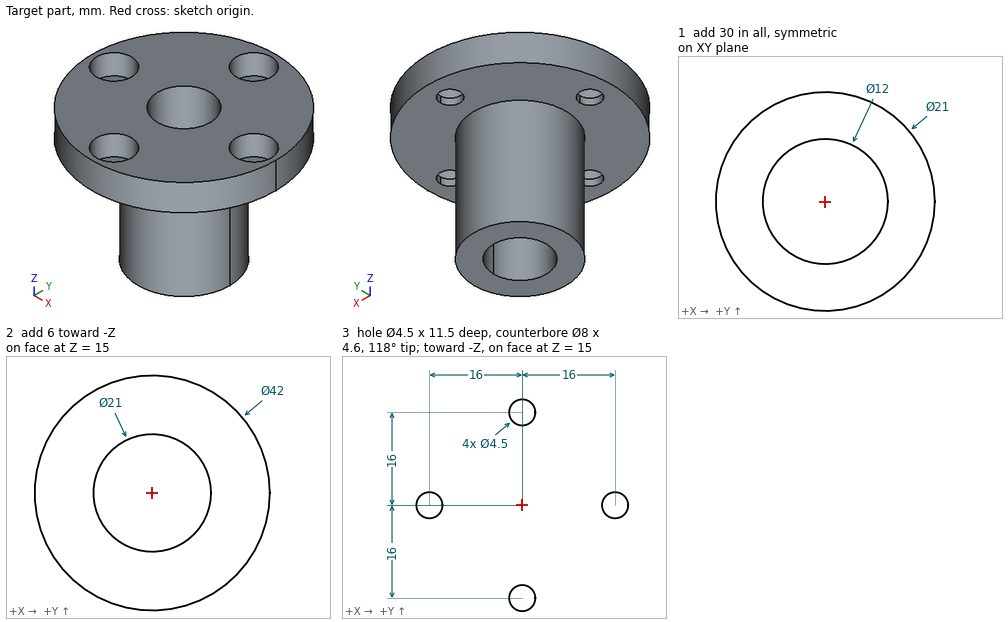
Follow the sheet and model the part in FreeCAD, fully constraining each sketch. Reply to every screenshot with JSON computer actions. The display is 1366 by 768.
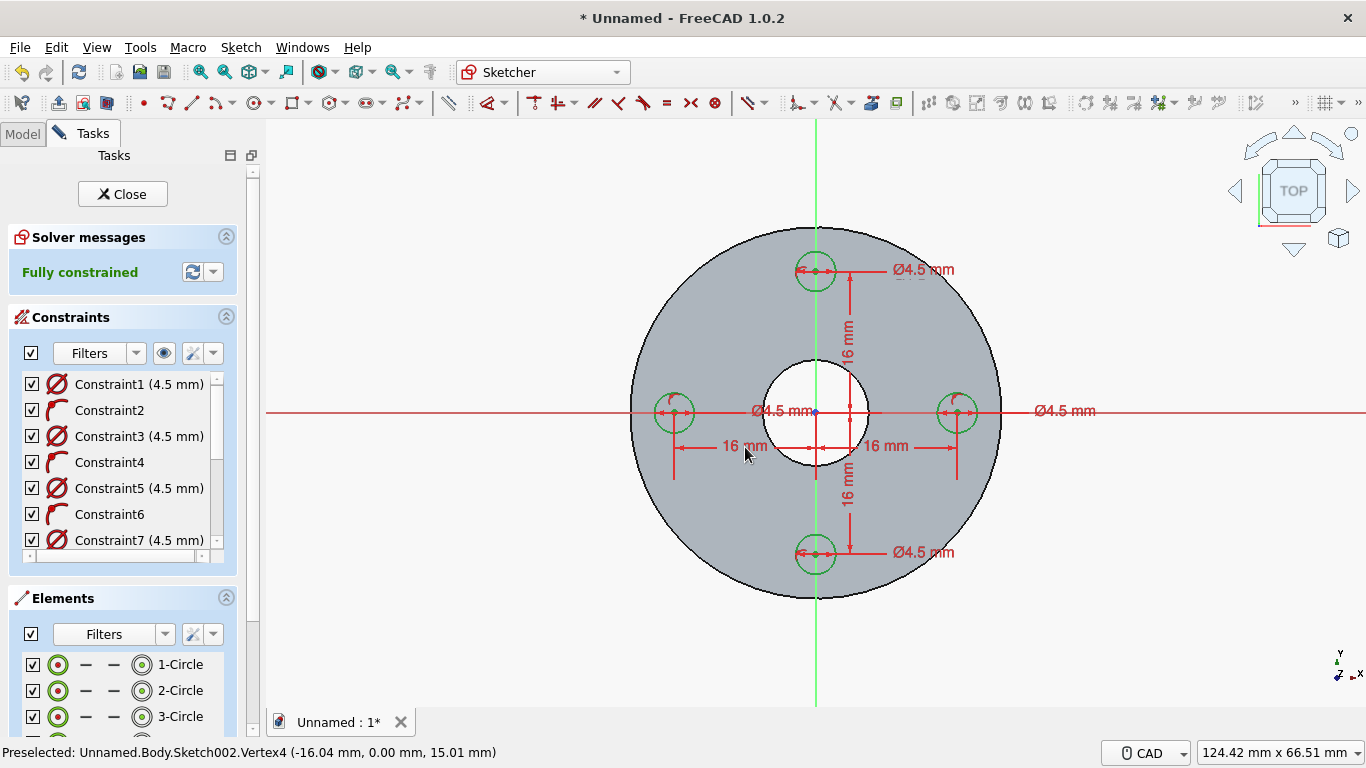
{"action": "left_click", "coordinate": [123, 194]}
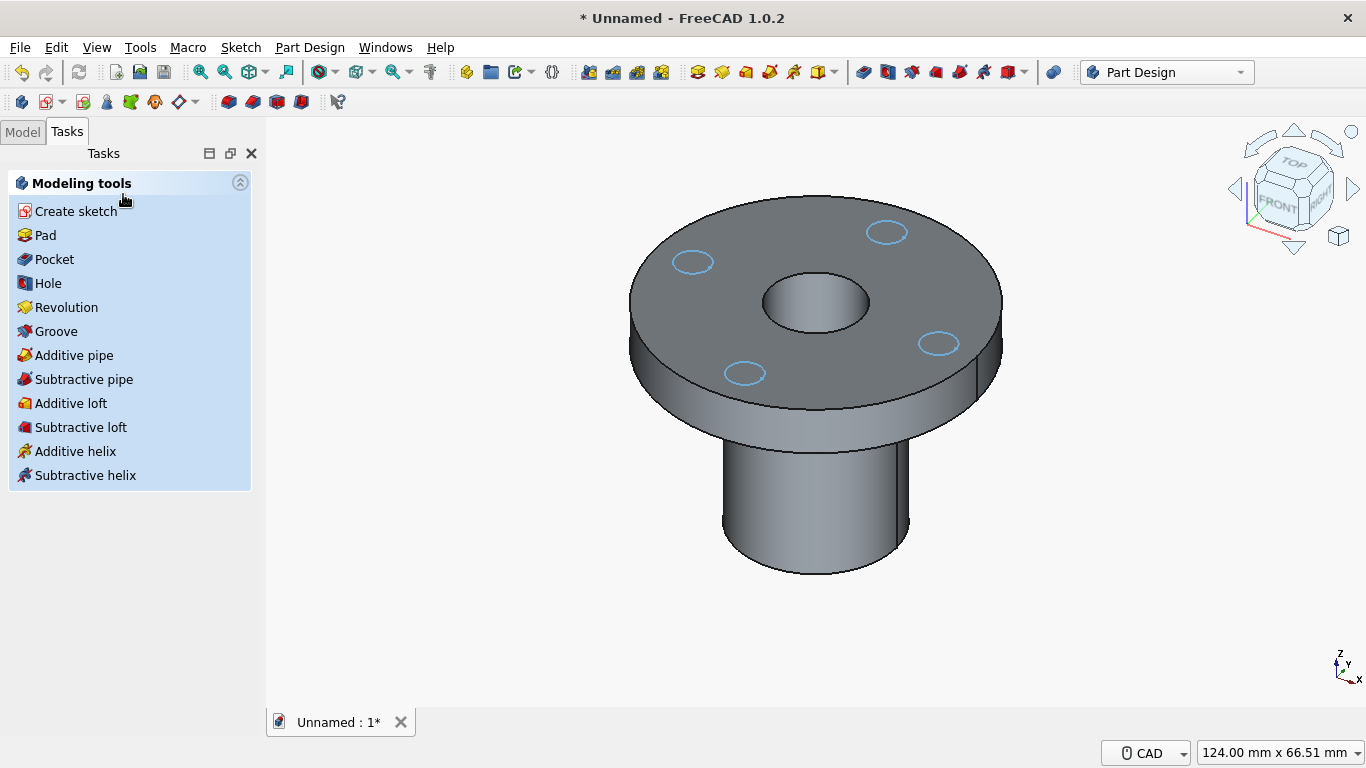
{"action": "left_click", "coordinate": [888, 72]}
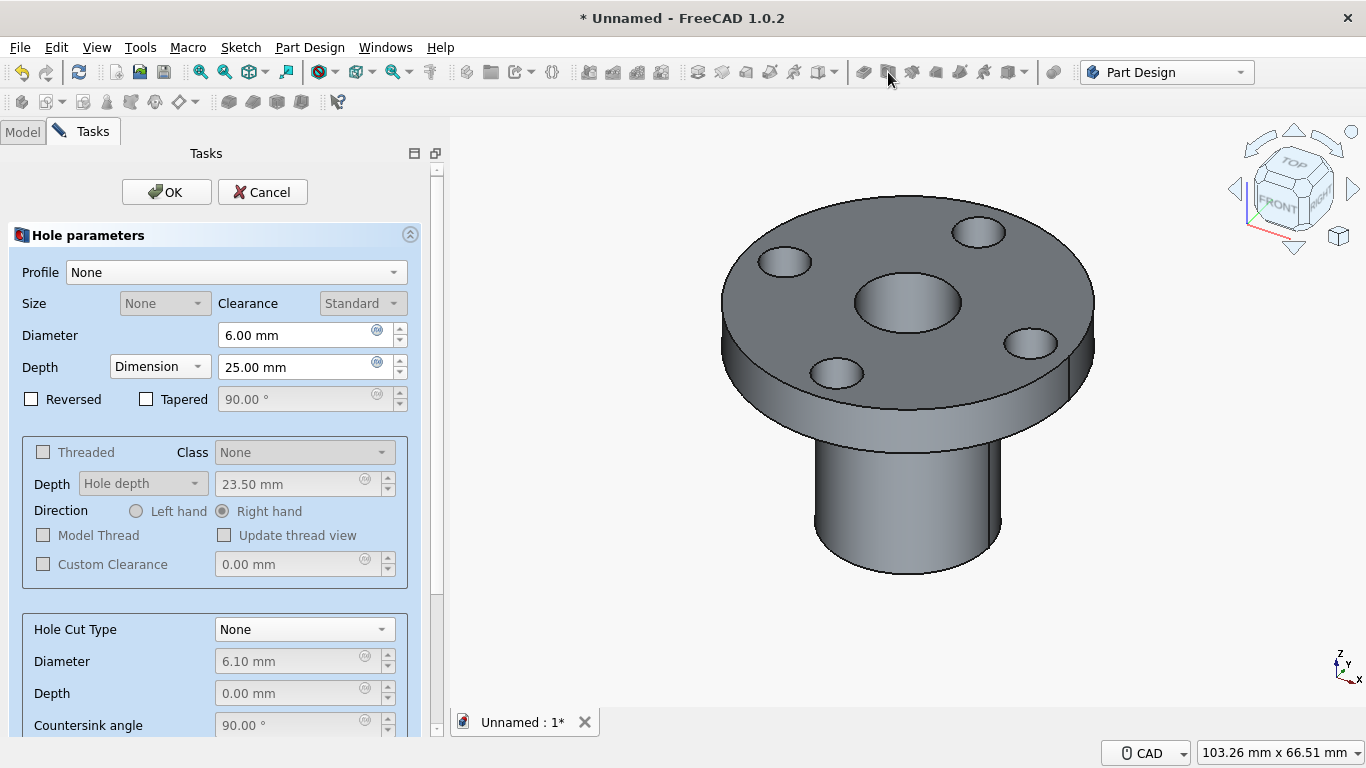
{"action": "triple_click", "coordinate": [305, 335]}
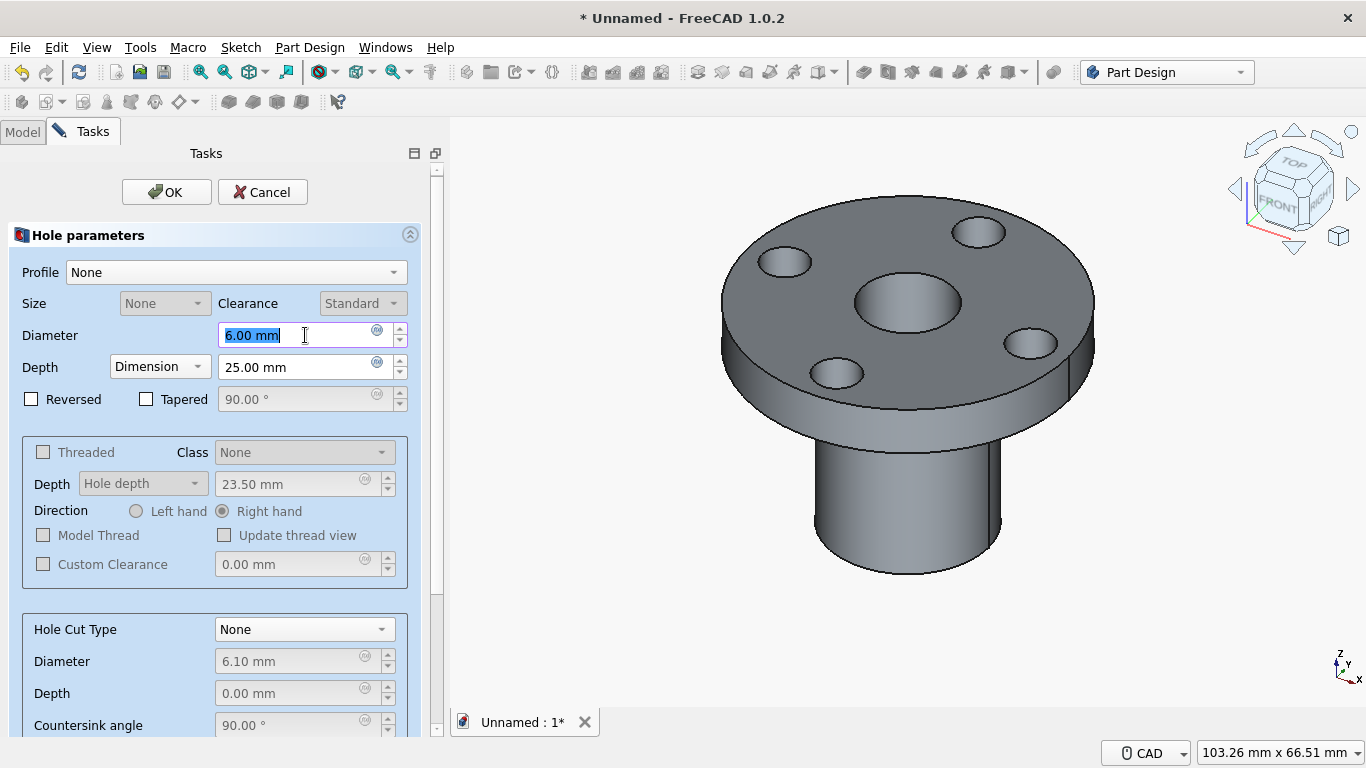
{"action": "type", "text": "4.5"}
{"action": "key", "text": "Tab"}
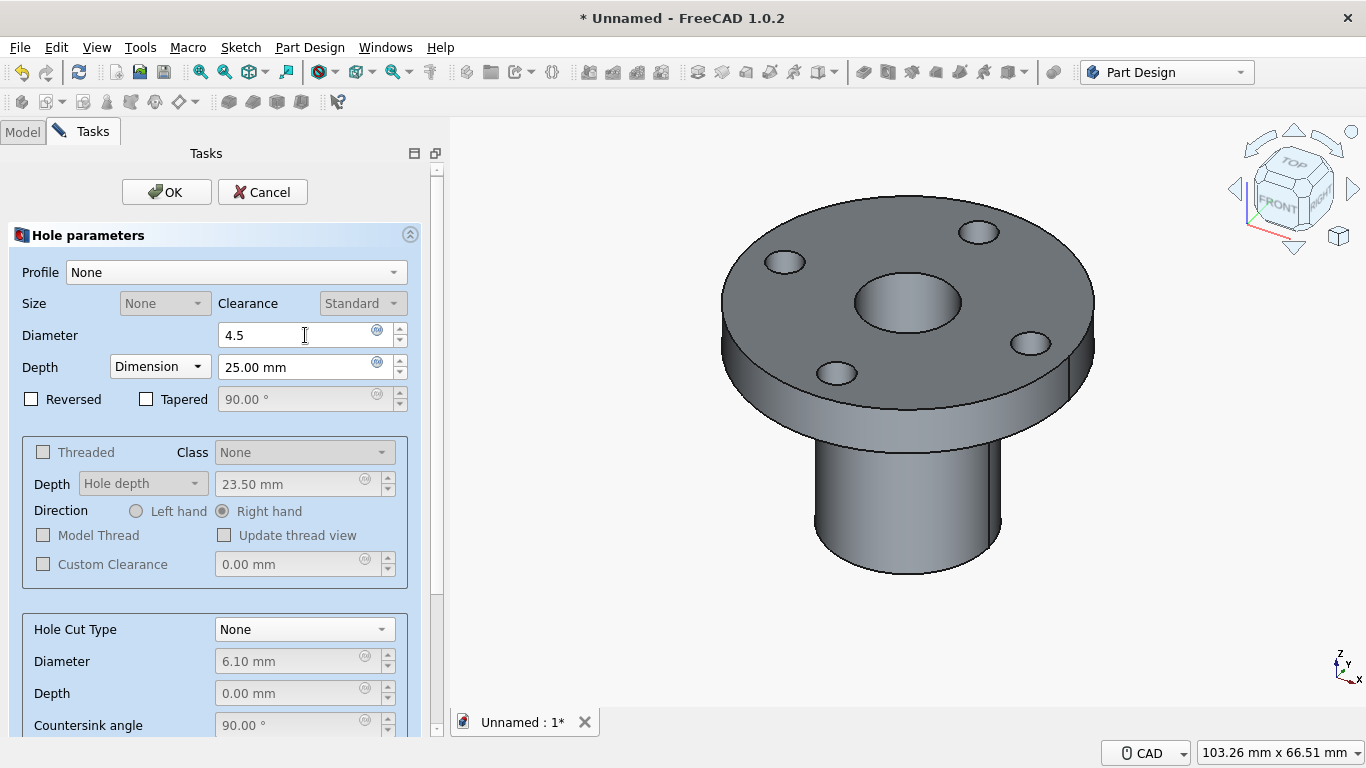
{"action": "triple_click", "coordinate": [305, 367]}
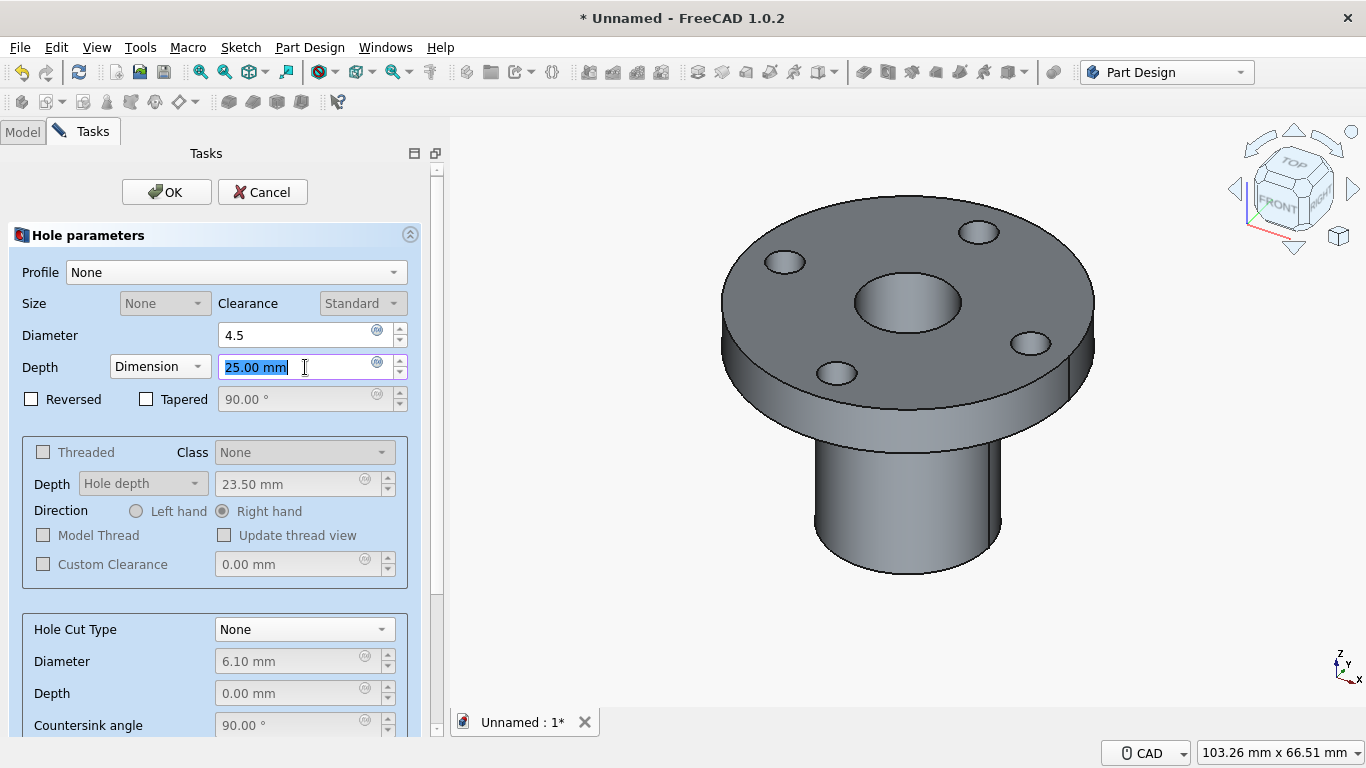
{"action": "type", "text": "11.5"}
{"action": "key", "text": "Tab"}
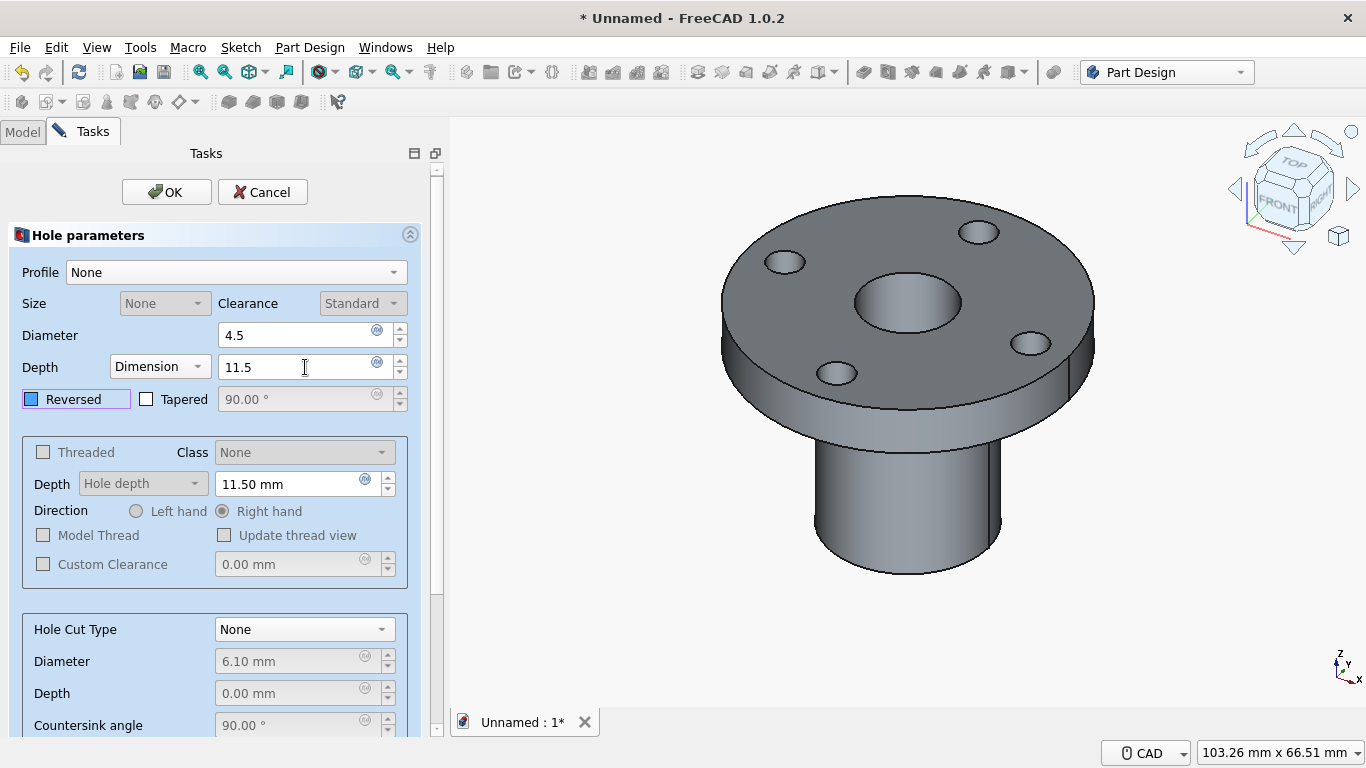
{"action": "left_click", "coordinate": [306, 630]}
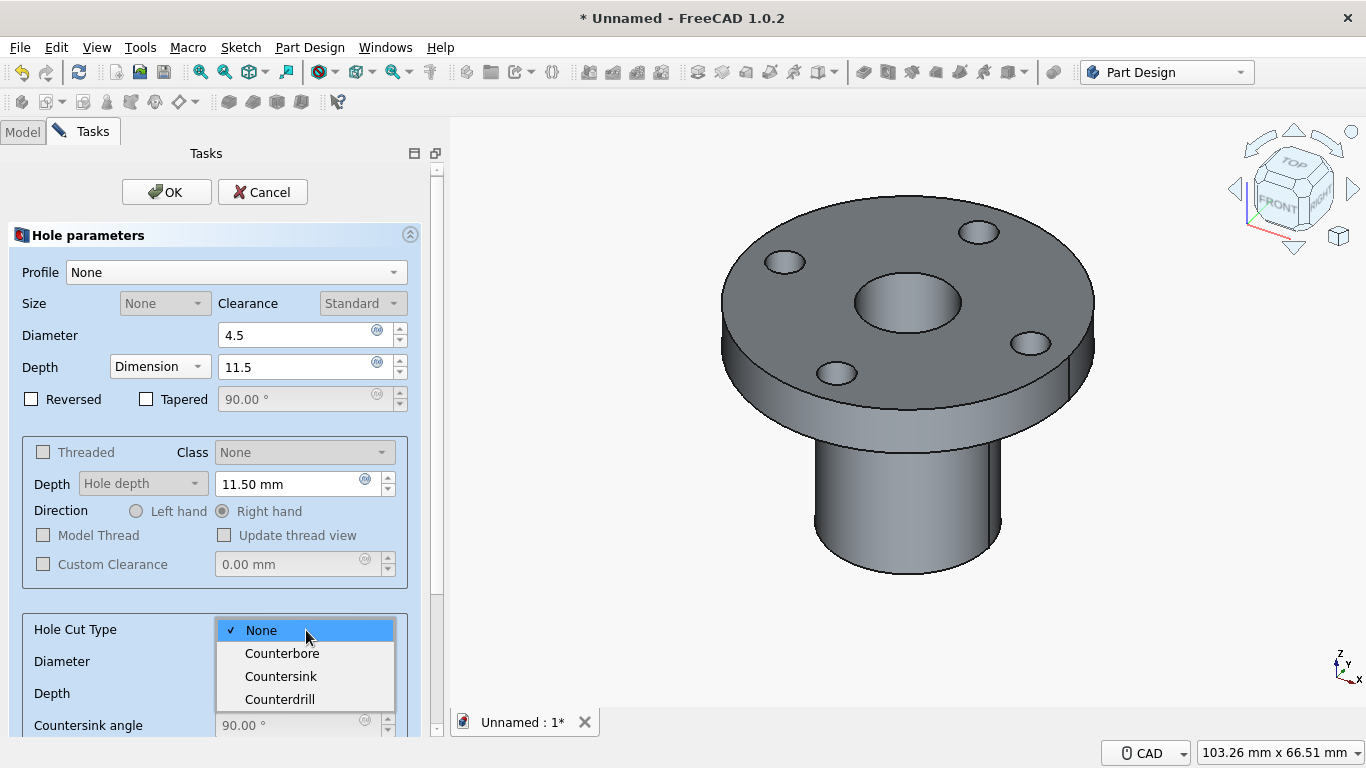
{"action": "left_click", "coordinate": [304, 654]}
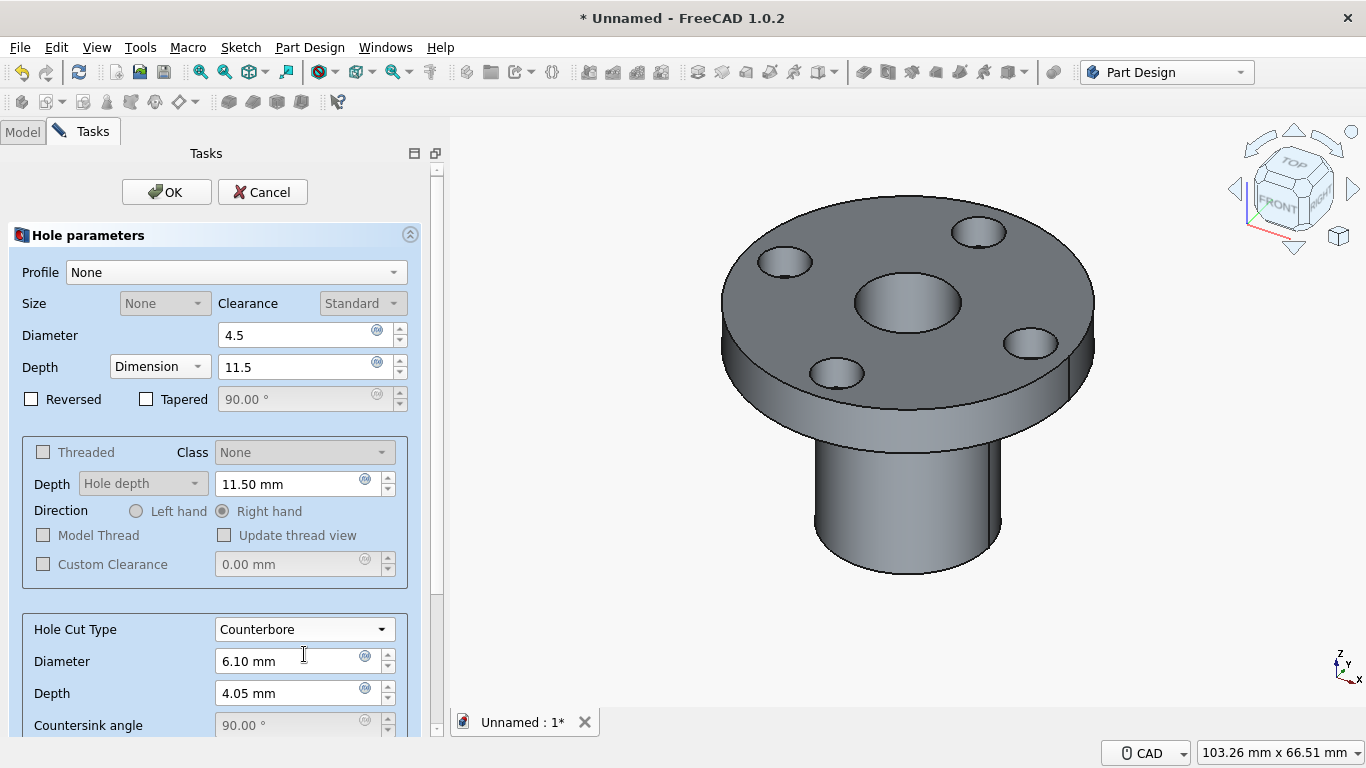
{"action": "triple_click", "coordinate": [298, 661]}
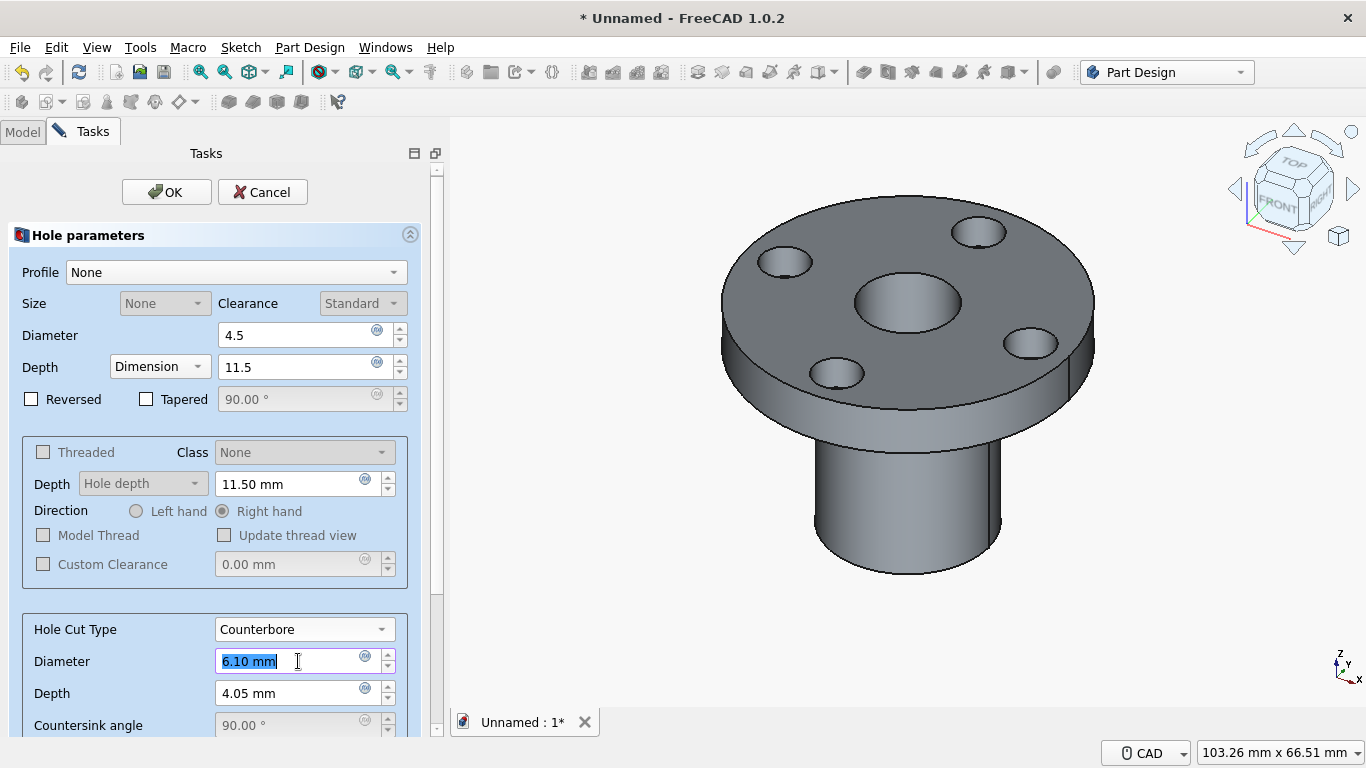
{"action": "type", "text": "8"}
{"action": "key", "text": "Tab"}